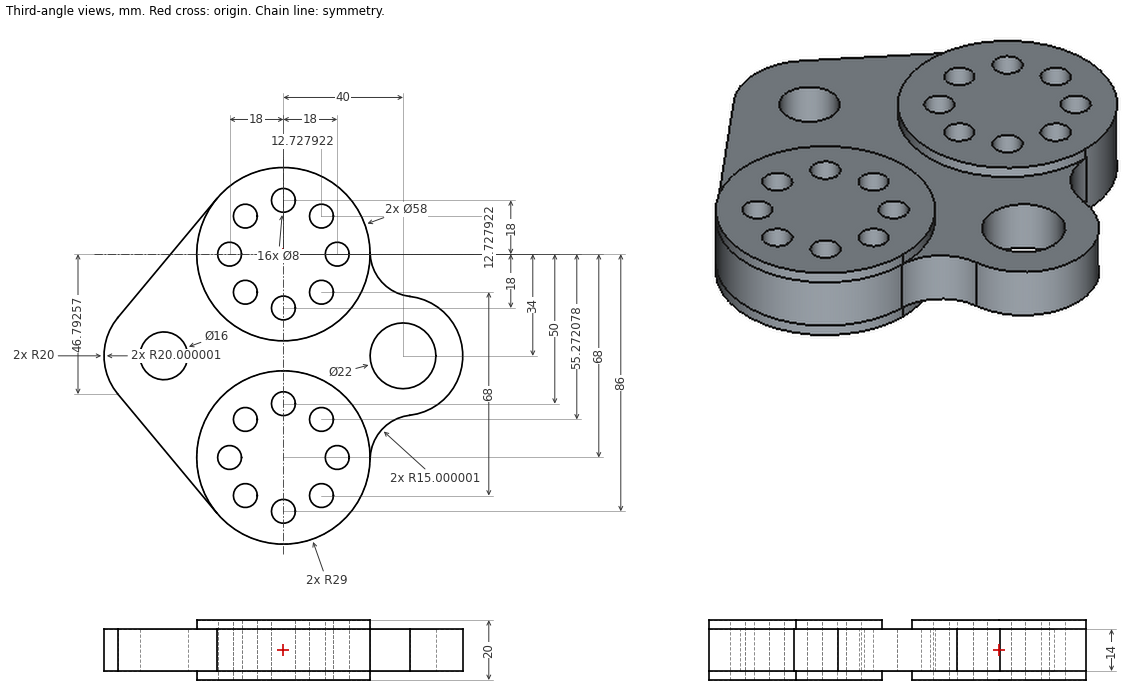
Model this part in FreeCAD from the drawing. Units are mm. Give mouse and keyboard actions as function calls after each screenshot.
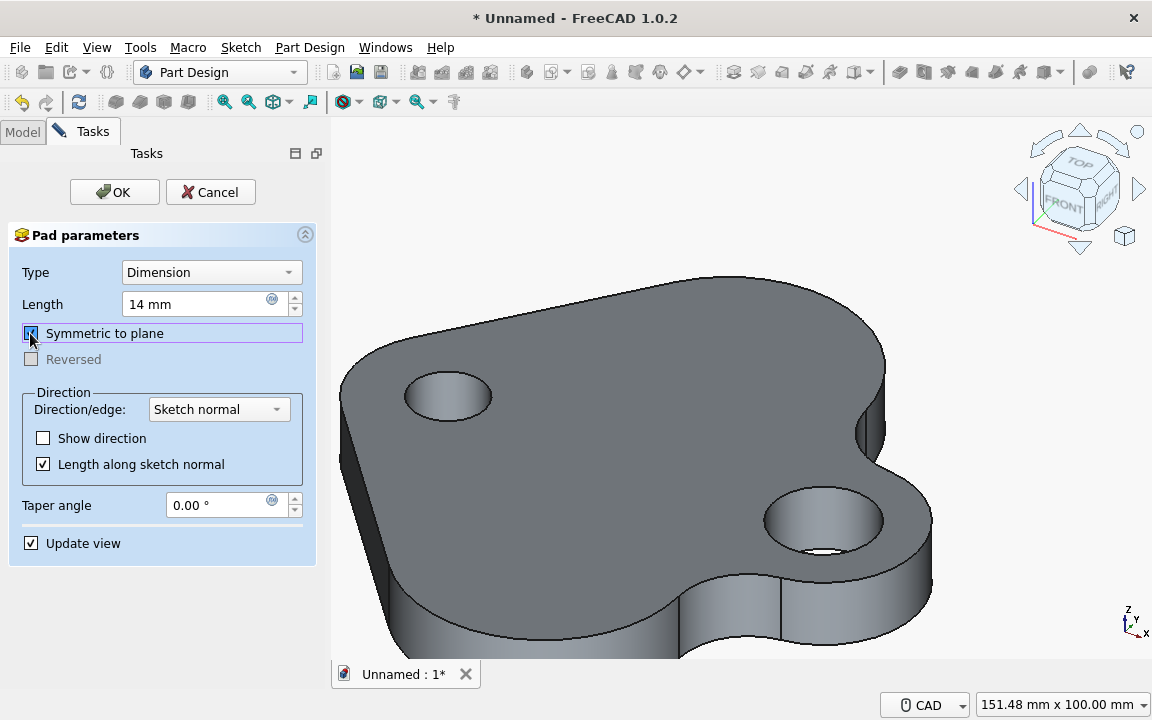
click(115, 192)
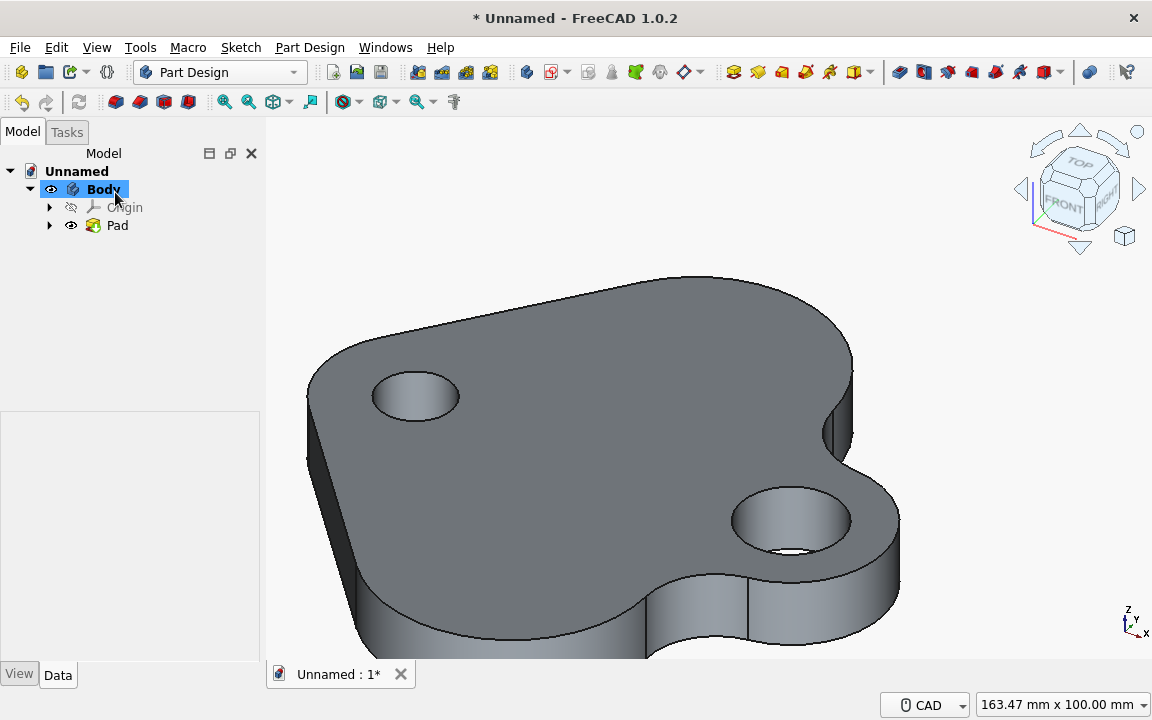
key(v)
key(f)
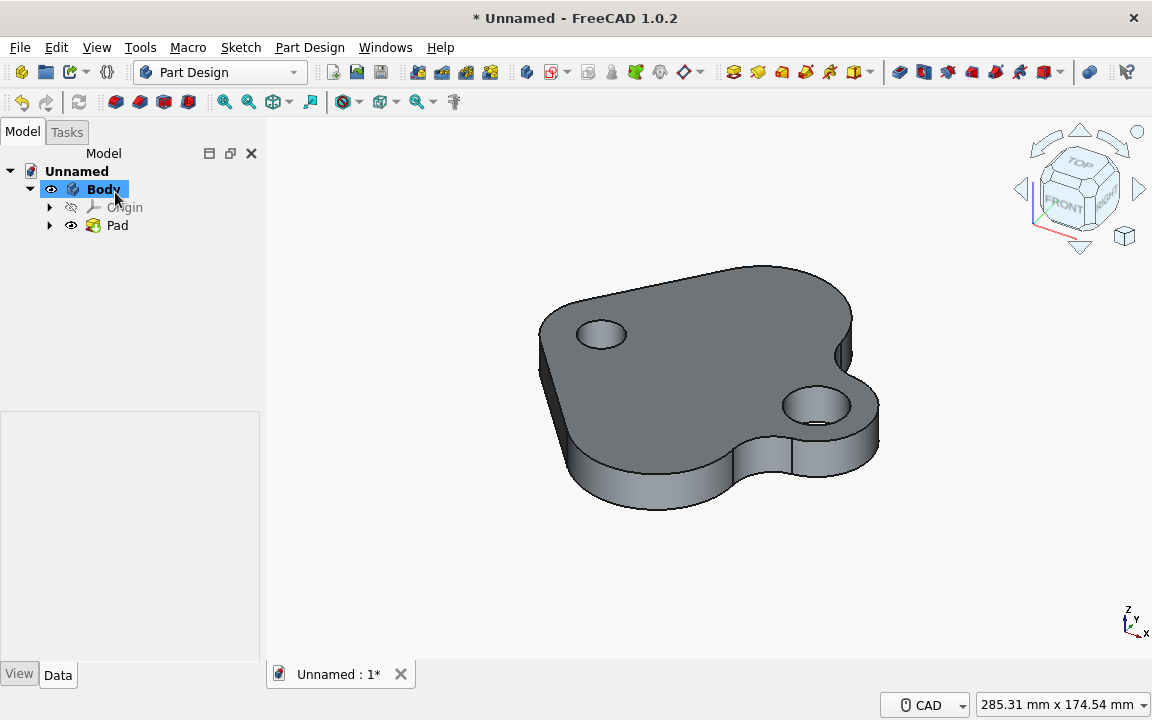
click(552, 72)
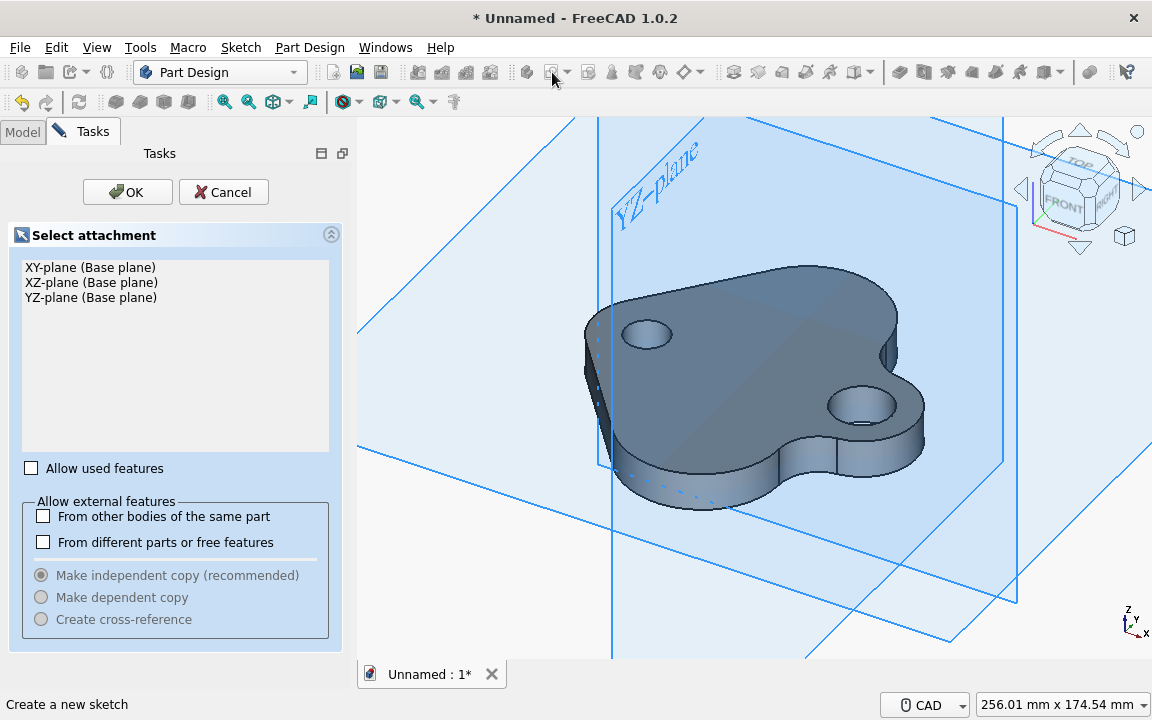
click(82, 268)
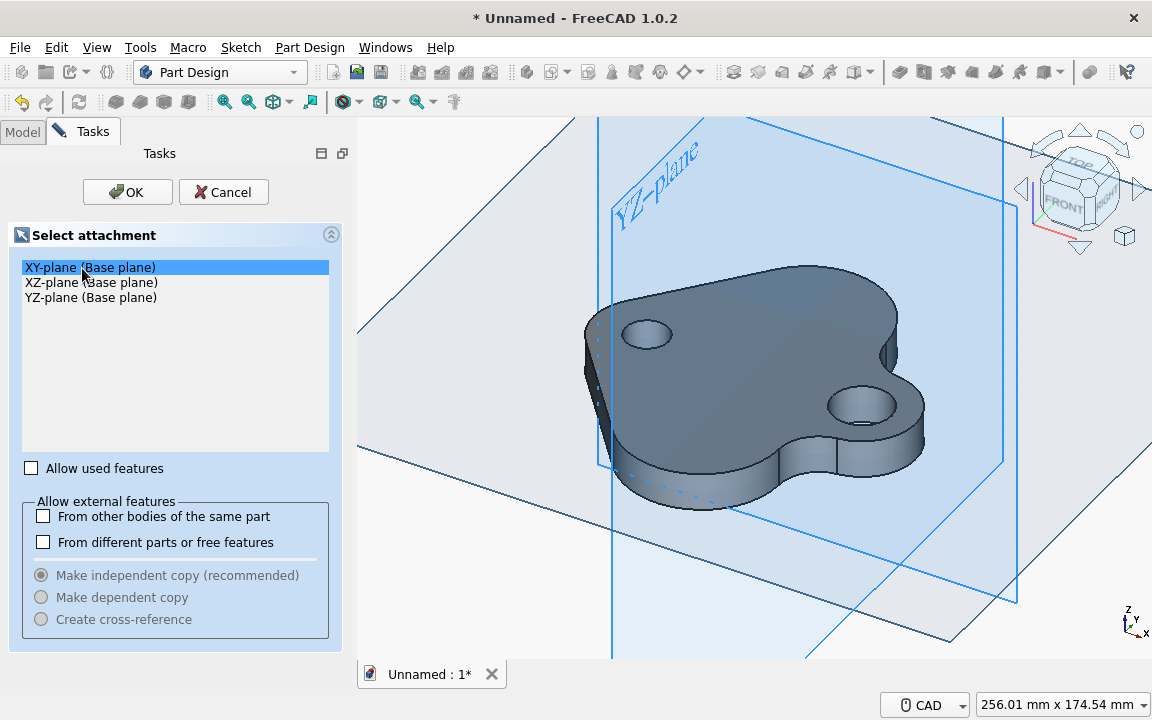
click(128, 192)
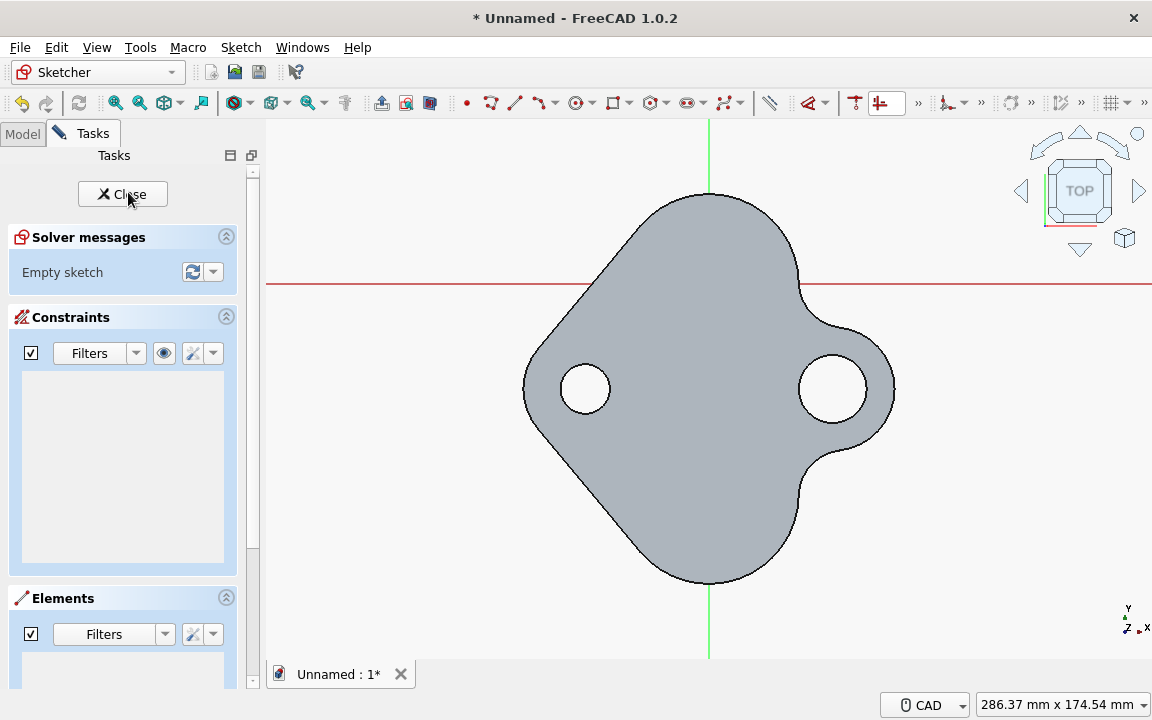
key(q)
key(s)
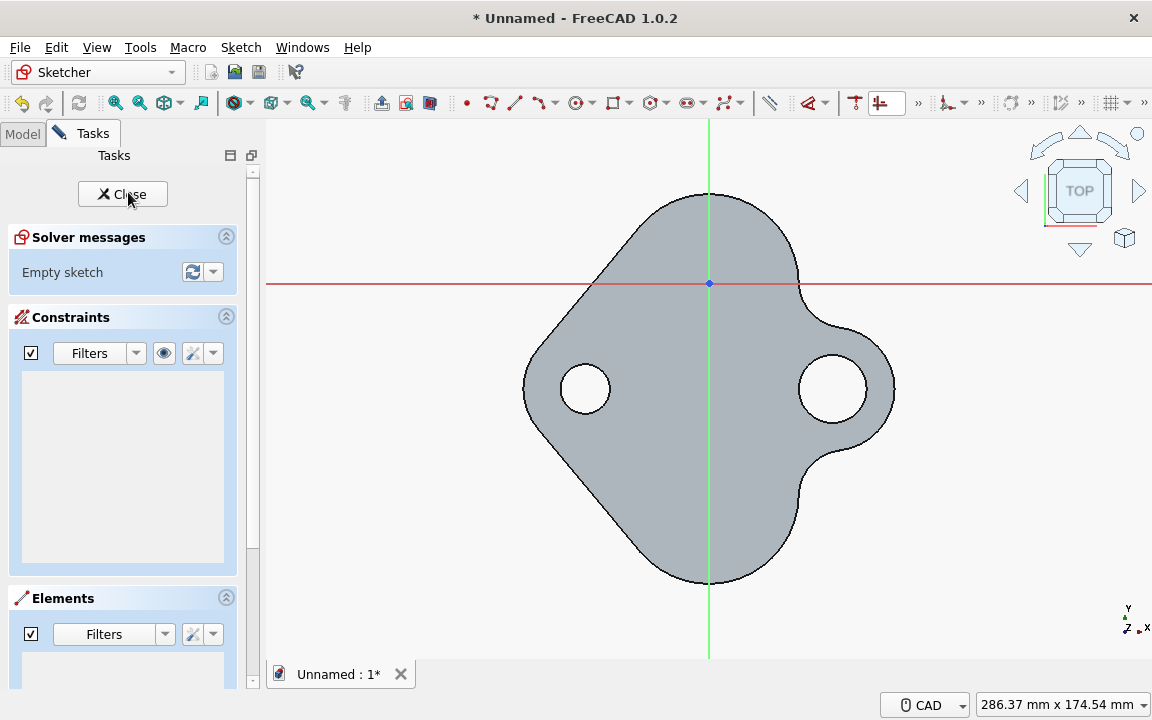
click(576, 104)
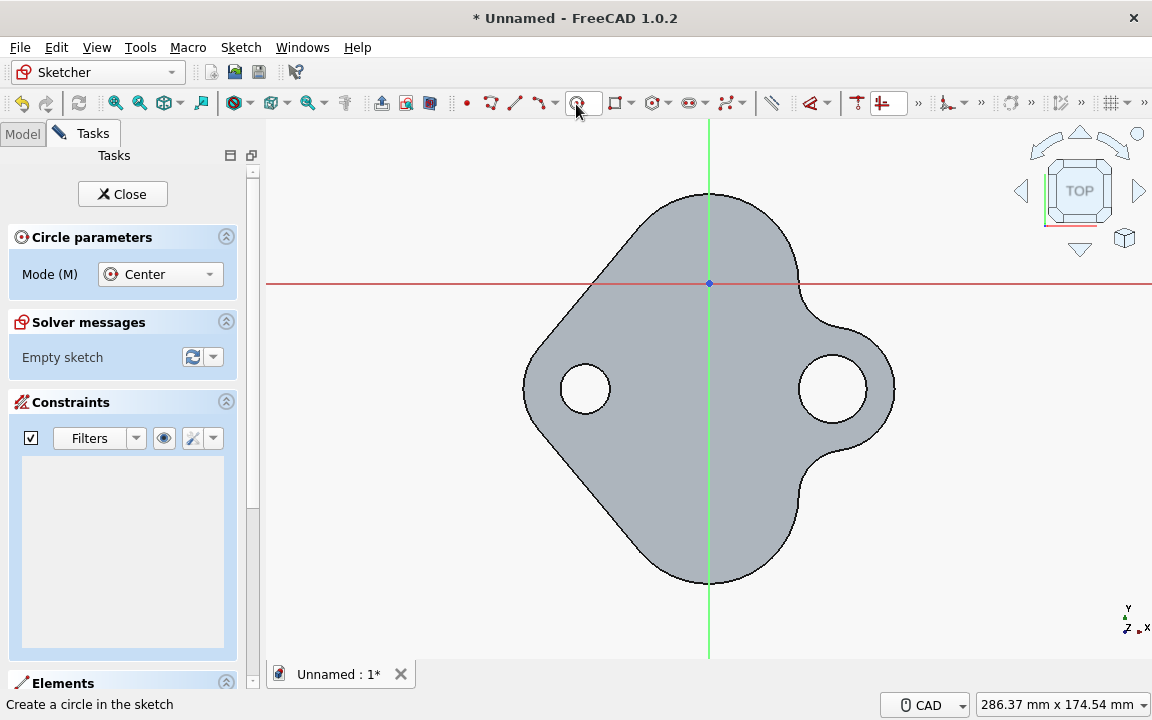
click(709, 284)
move(772, 220)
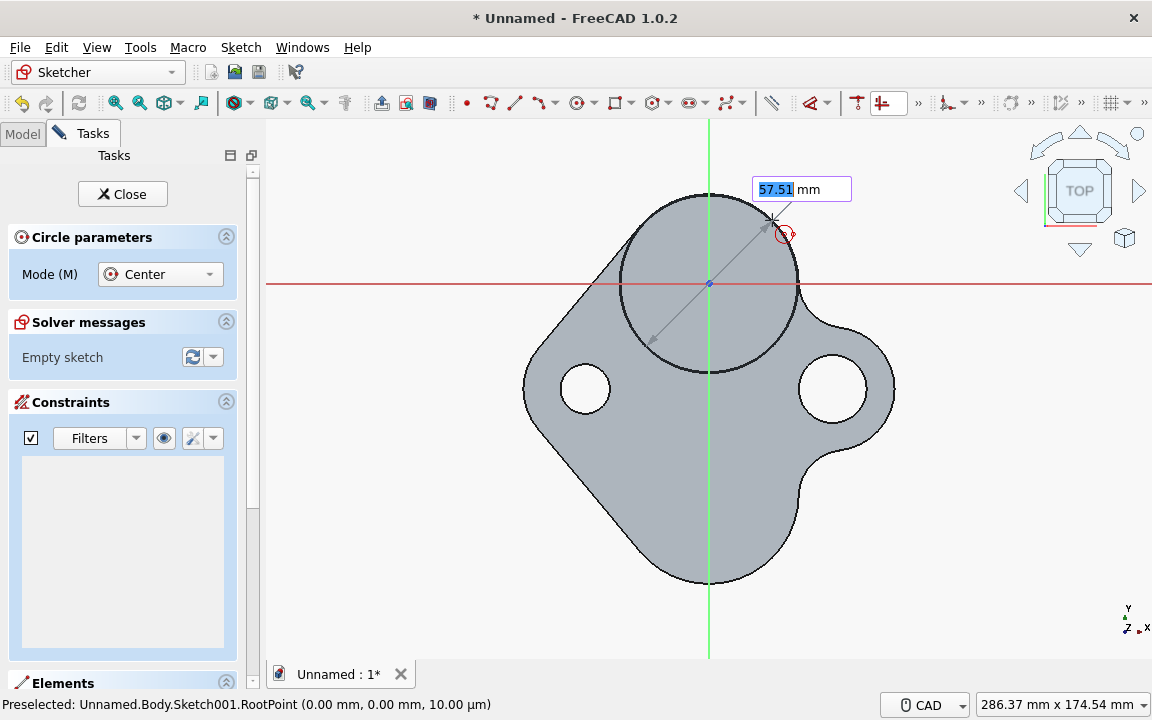
text(58)
key(Return)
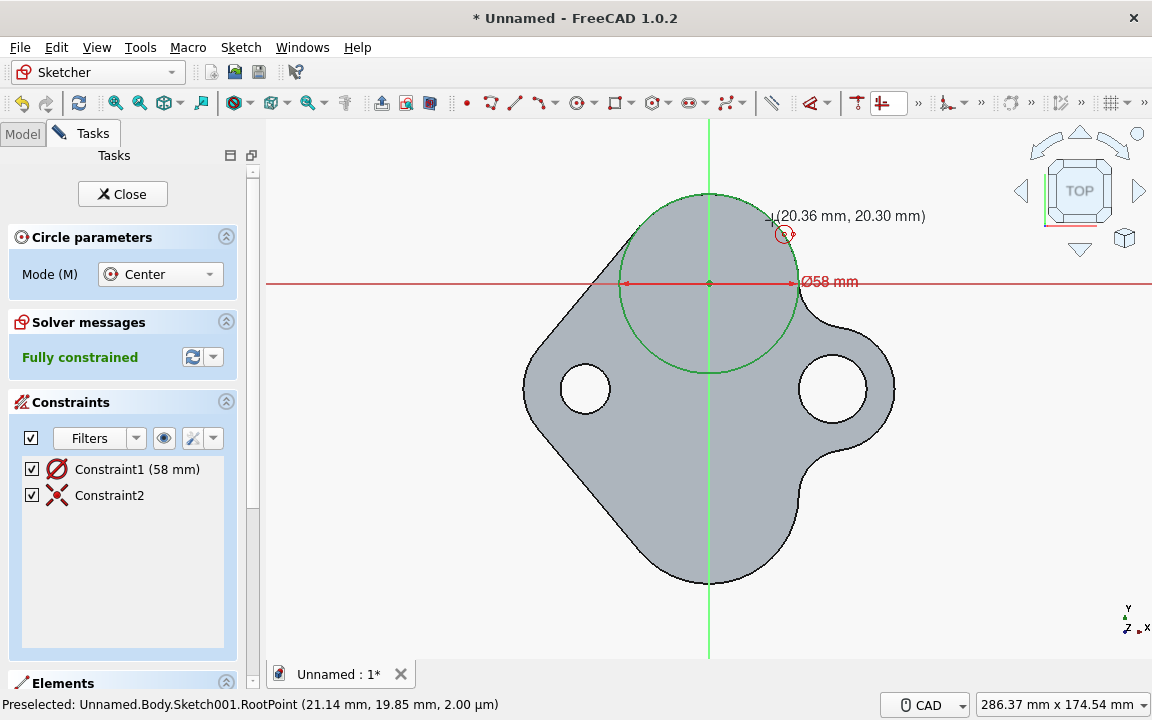
click(709, 494)
move(772, 431)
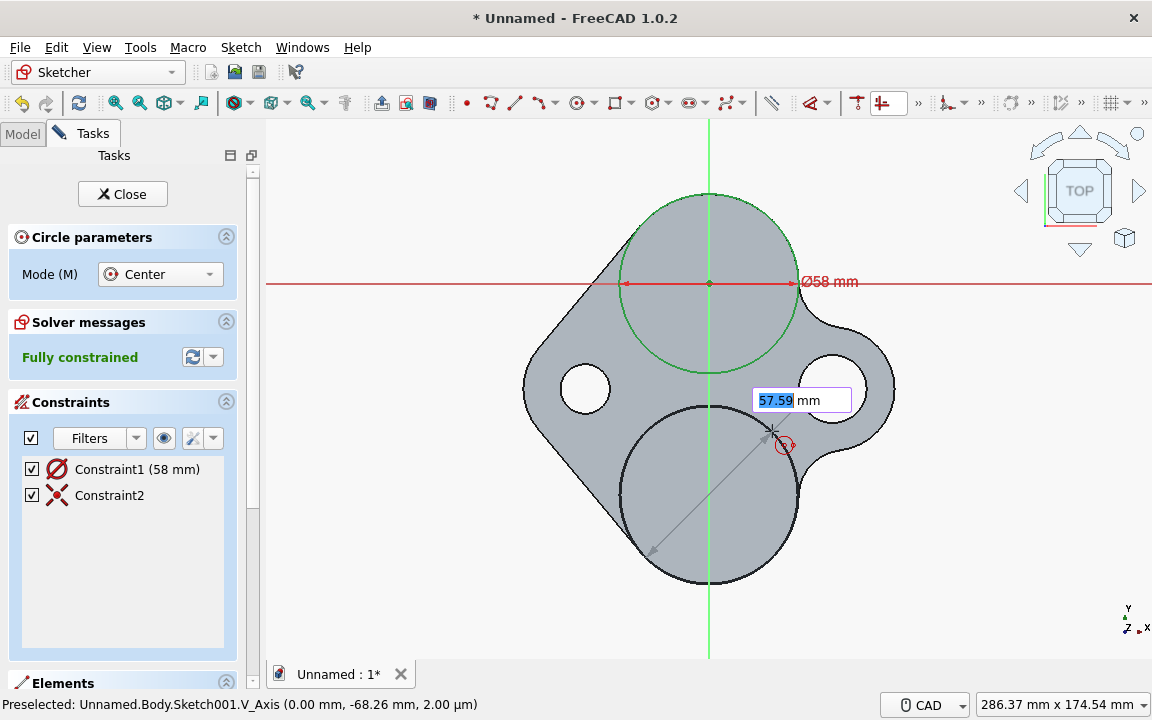
text(58)
key(Return)
key(Escape)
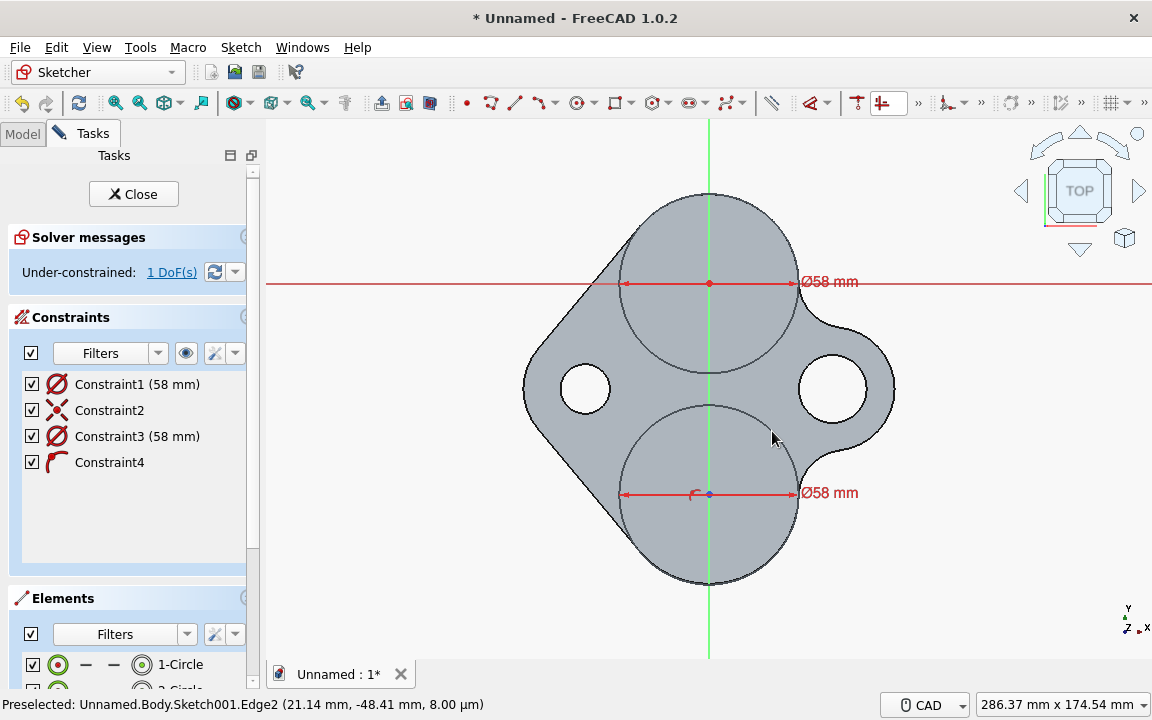
click(709, 495)